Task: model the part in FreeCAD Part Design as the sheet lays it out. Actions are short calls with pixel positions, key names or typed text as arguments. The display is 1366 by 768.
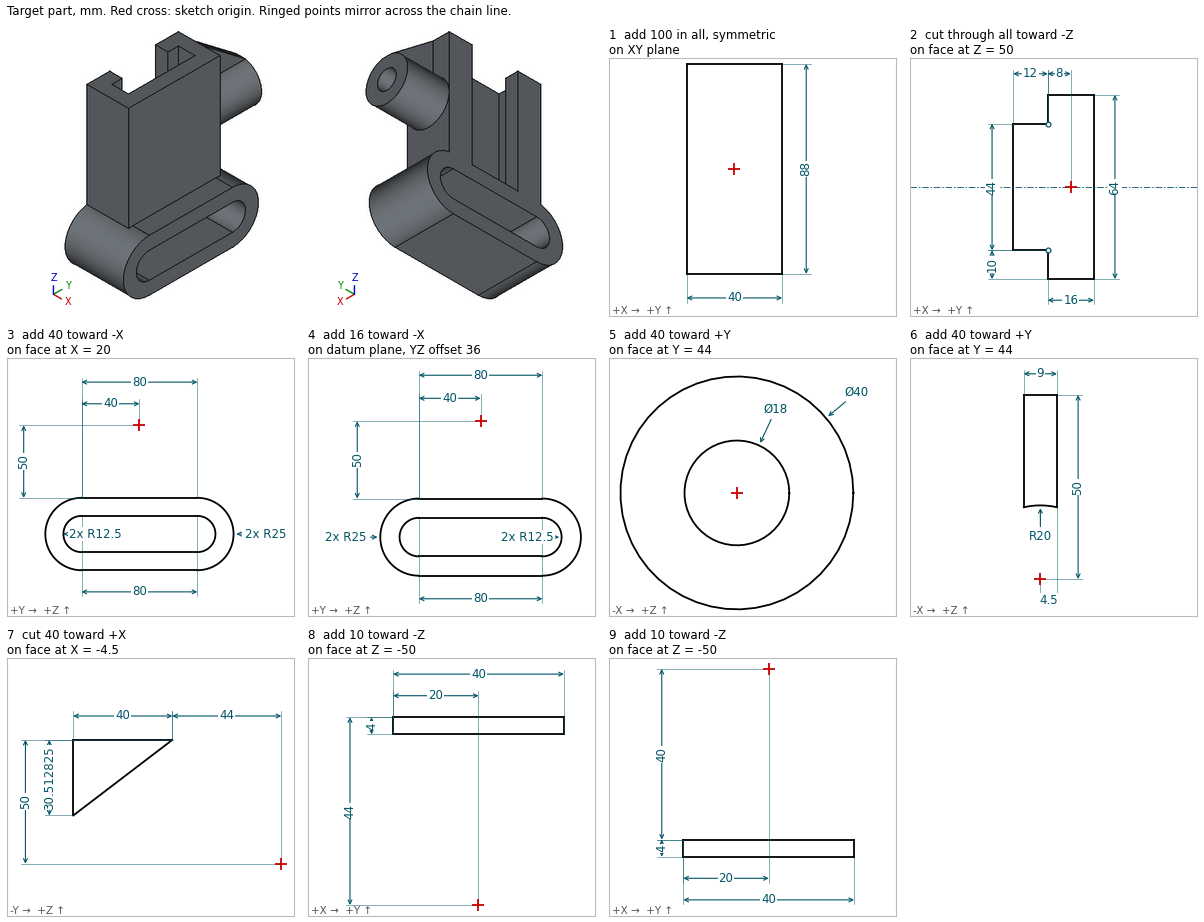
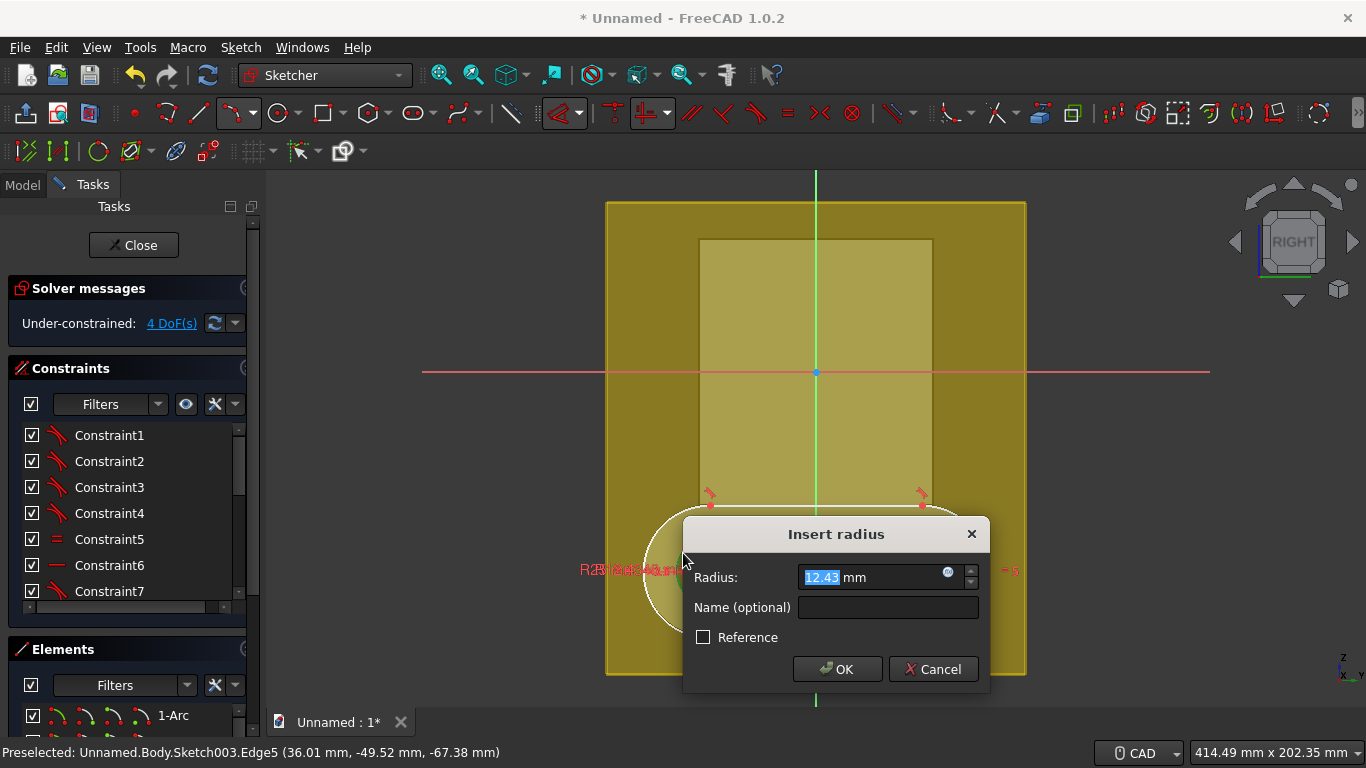
text(12.5)
key(Return)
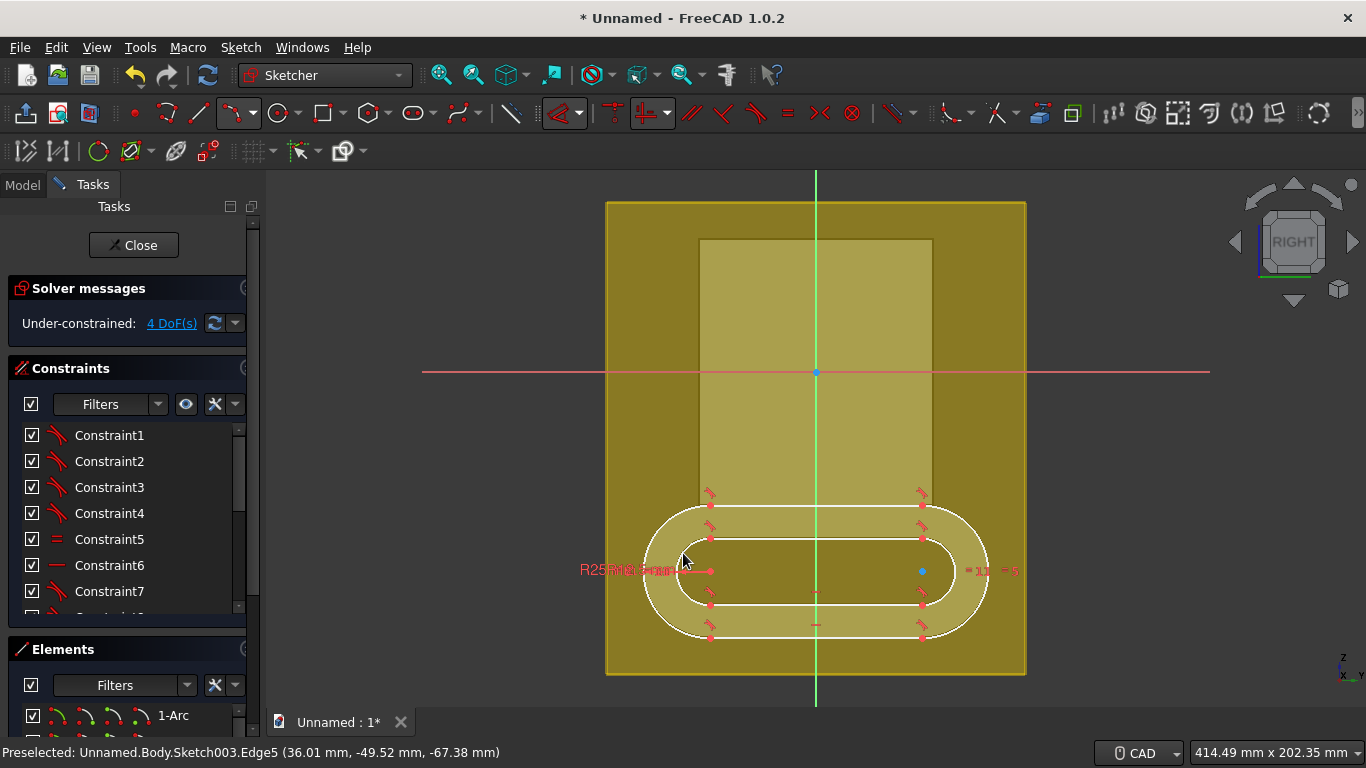
click(774, 506)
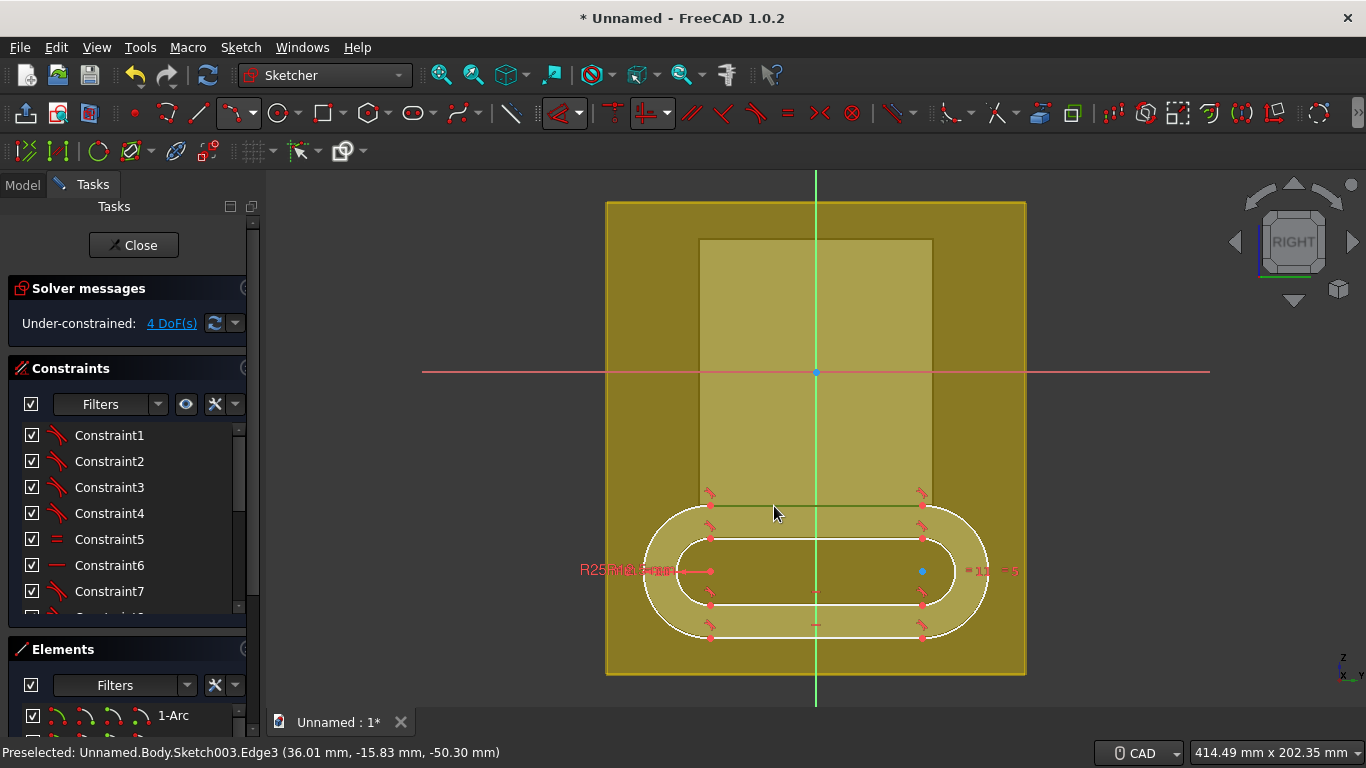
key(l)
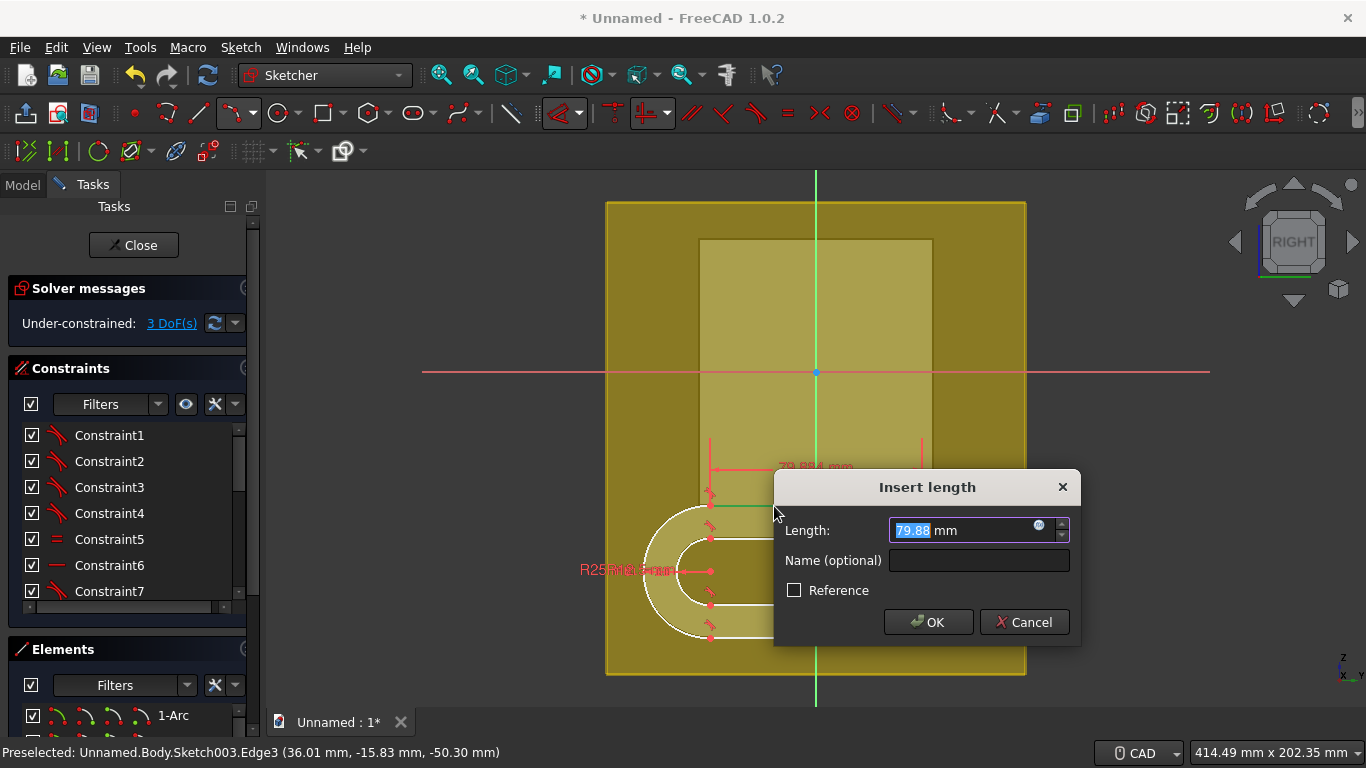
text(80)
key(Return)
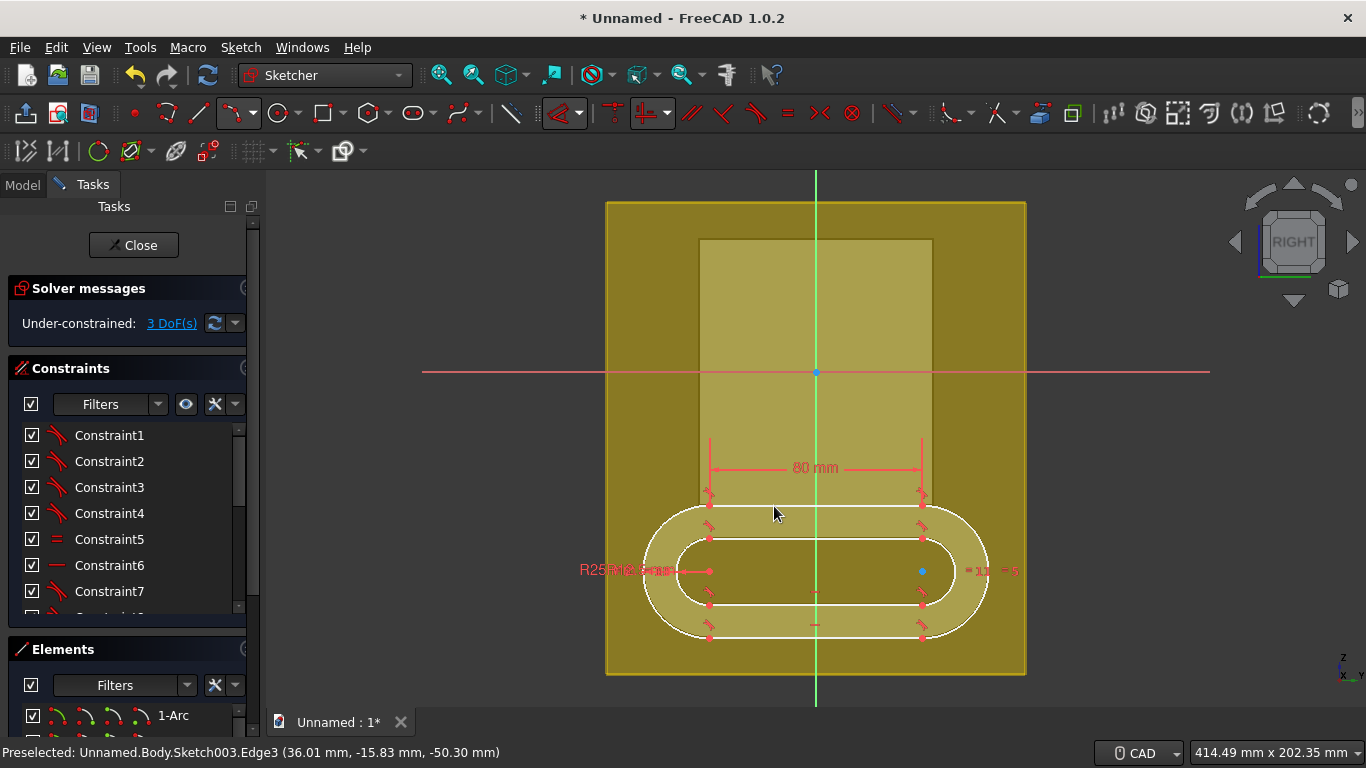
click(773, 539)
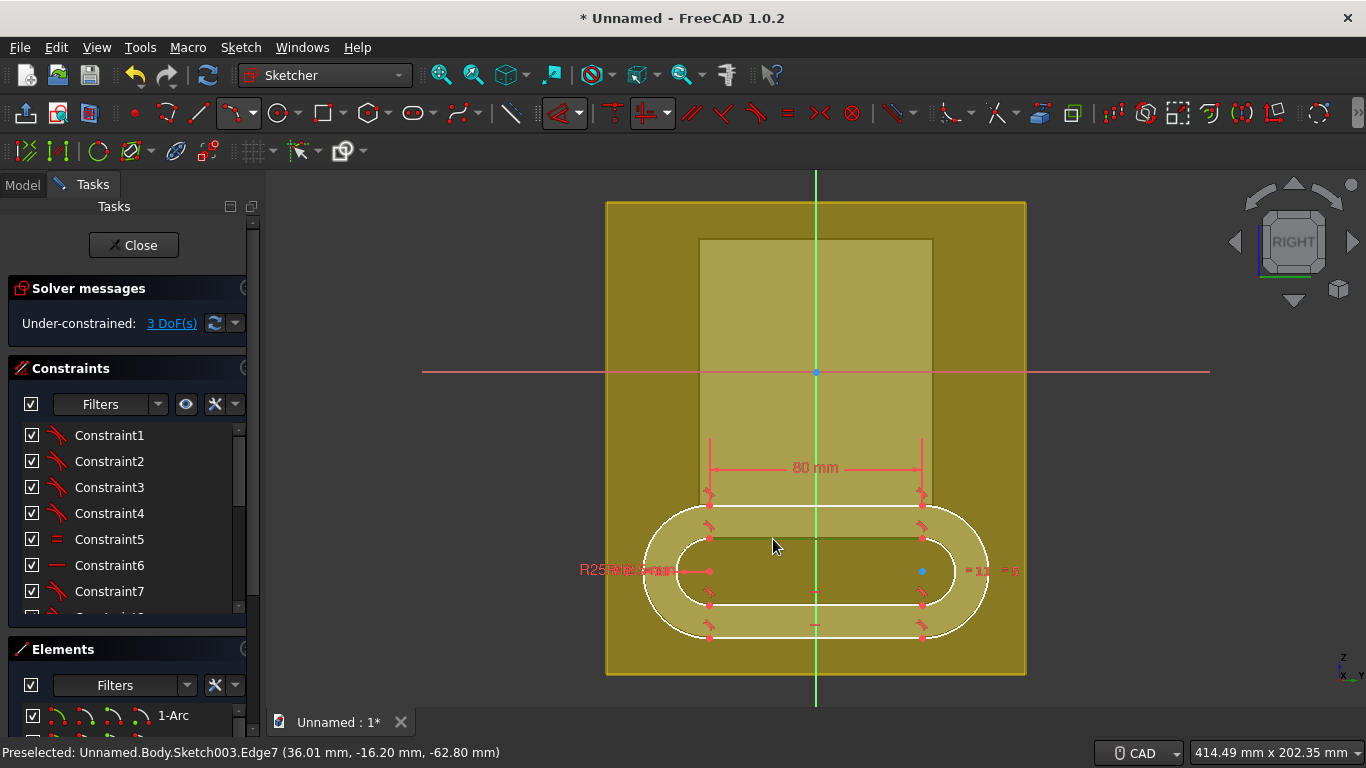
key(l)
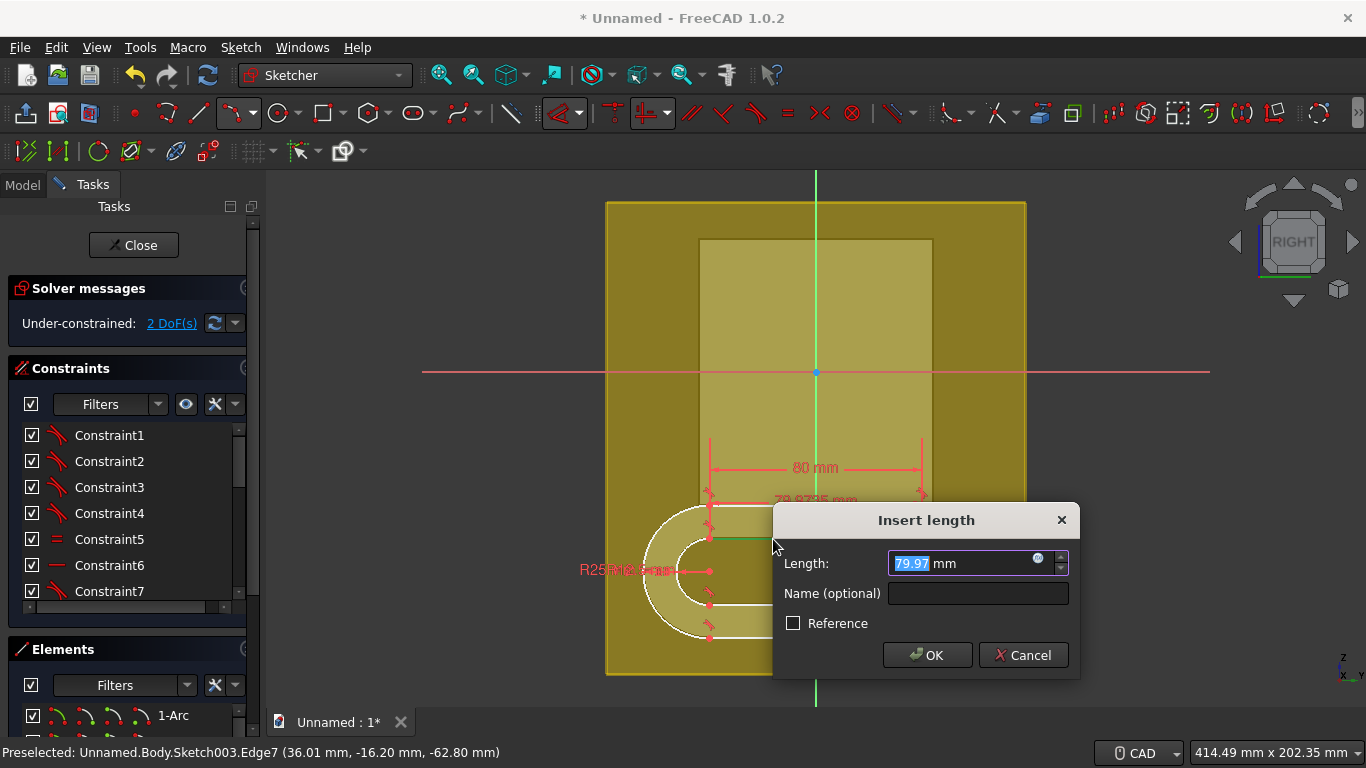
text(80)
key(Return)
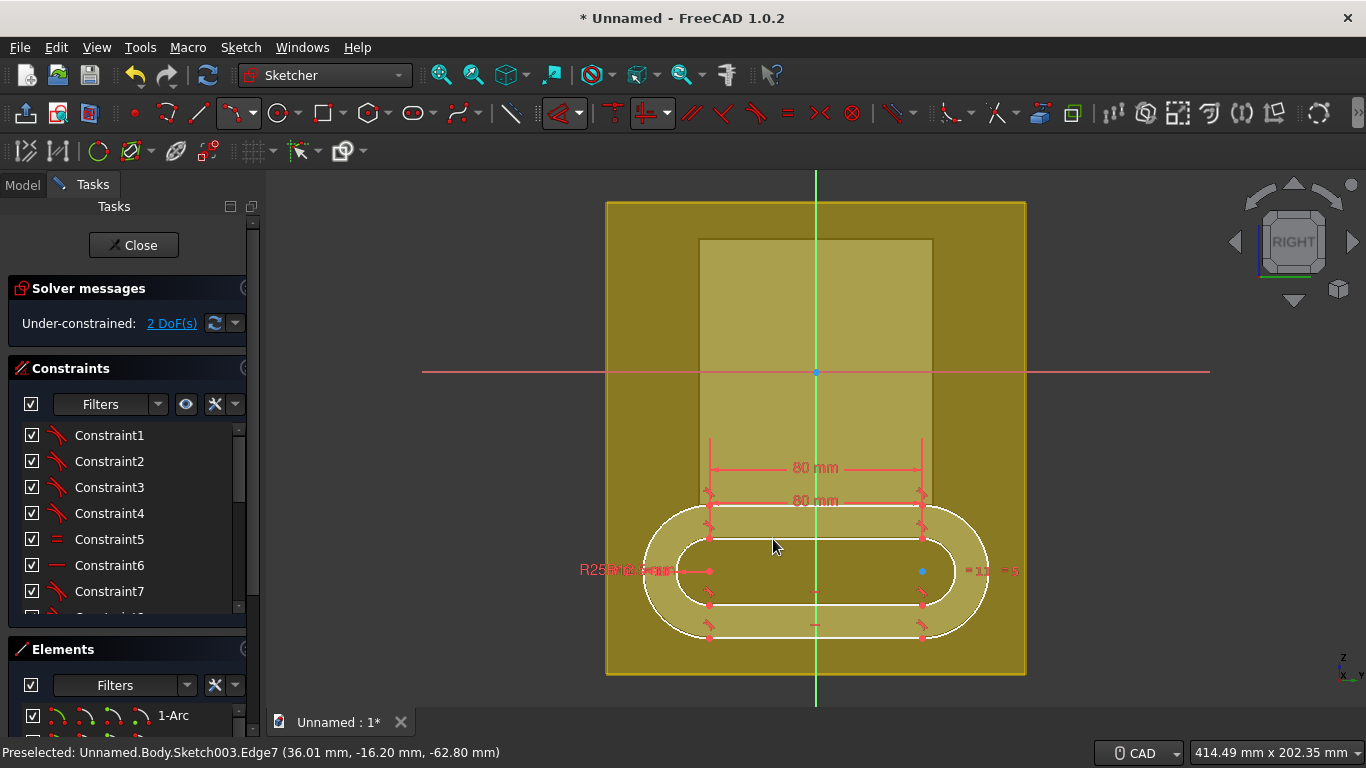
click(710, 506)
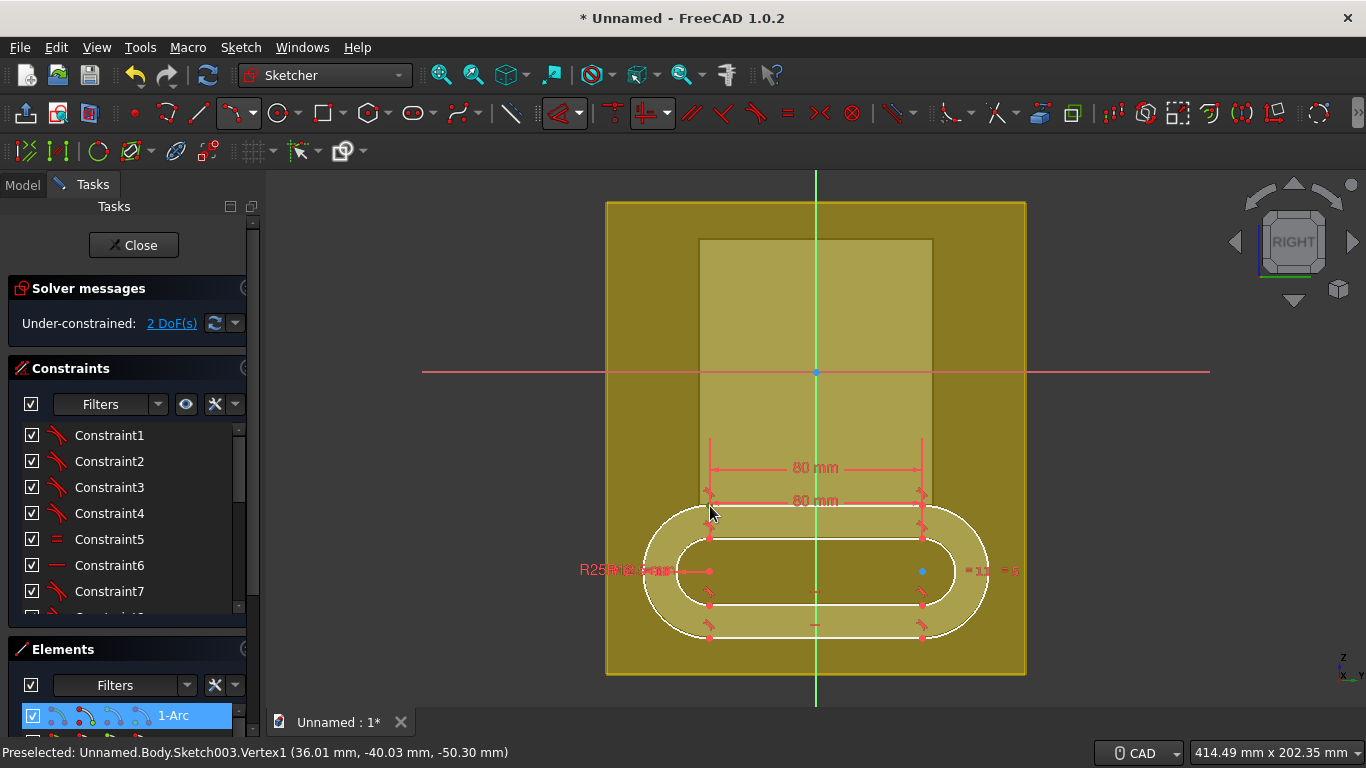
key(l)